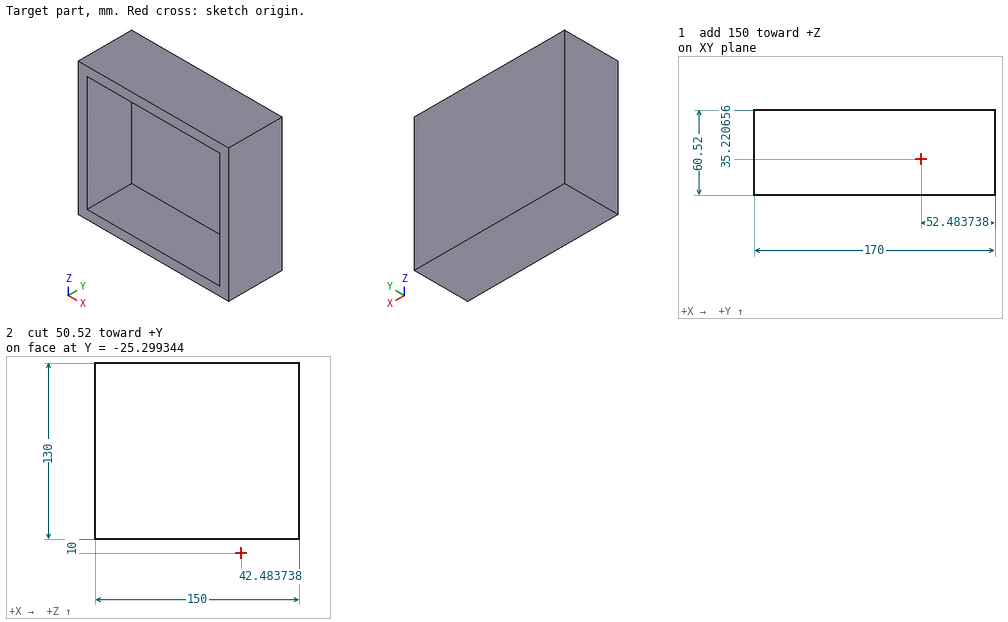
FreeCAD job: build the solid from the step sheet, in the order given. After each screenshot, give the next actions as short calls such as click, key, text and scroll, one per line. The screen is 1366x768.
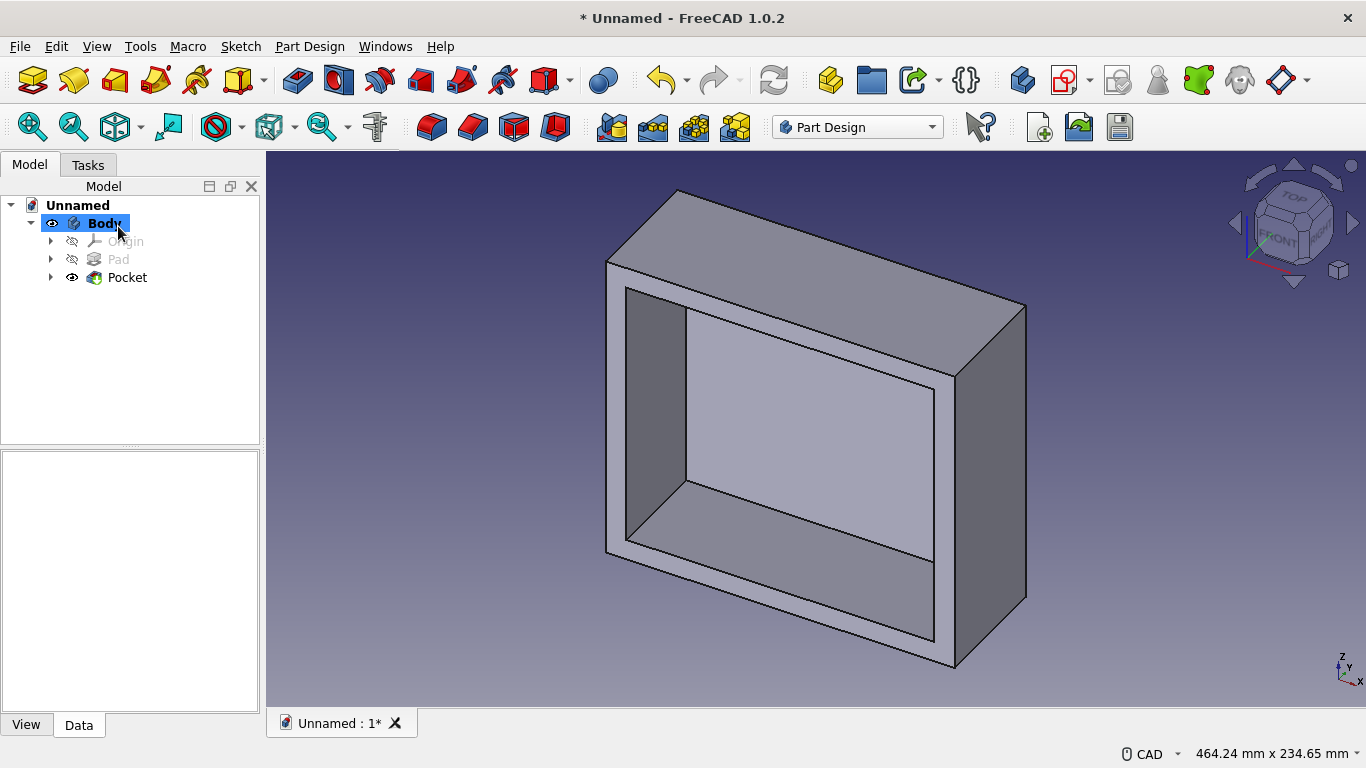
key(0)